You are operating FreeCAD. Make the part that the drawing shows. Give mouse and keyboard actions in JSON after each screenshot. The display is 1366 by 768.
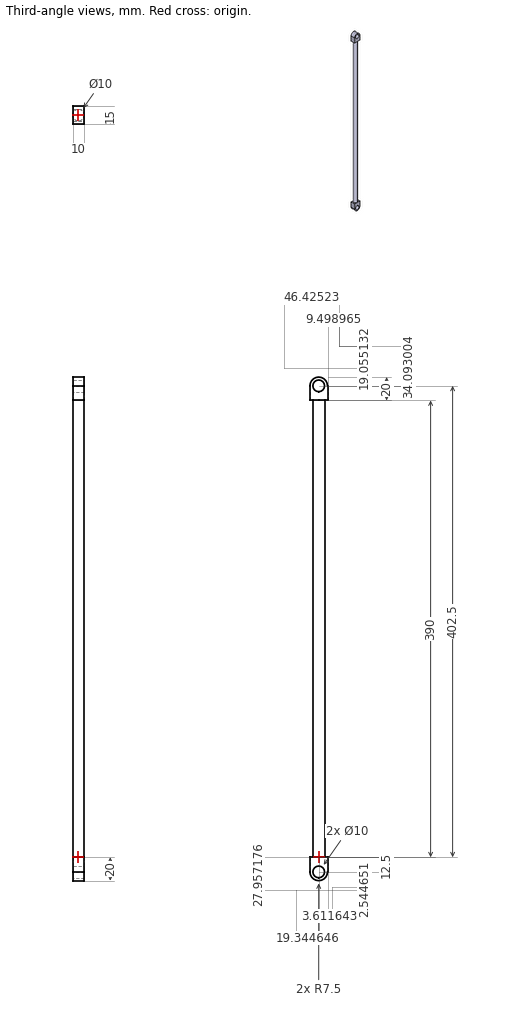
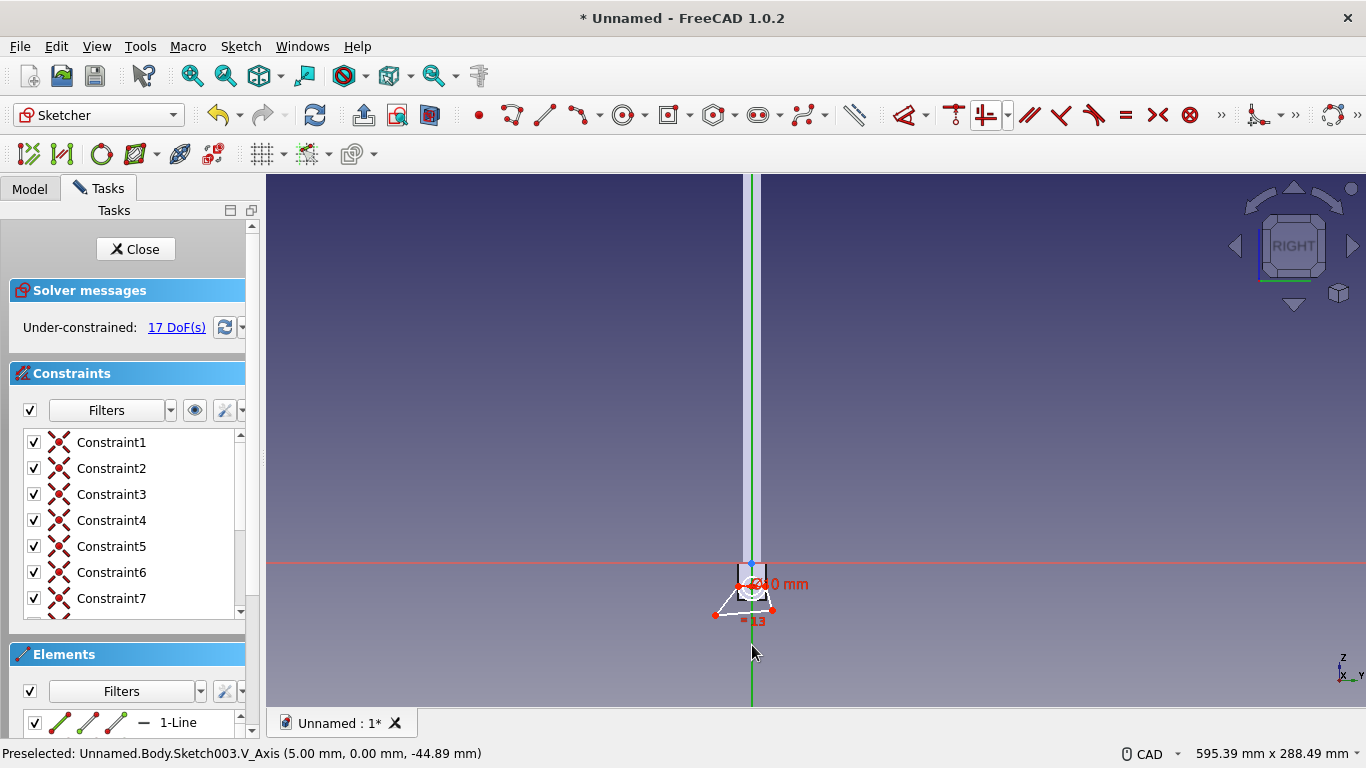
{"action": "left_click", "coordinate": [954, 116]}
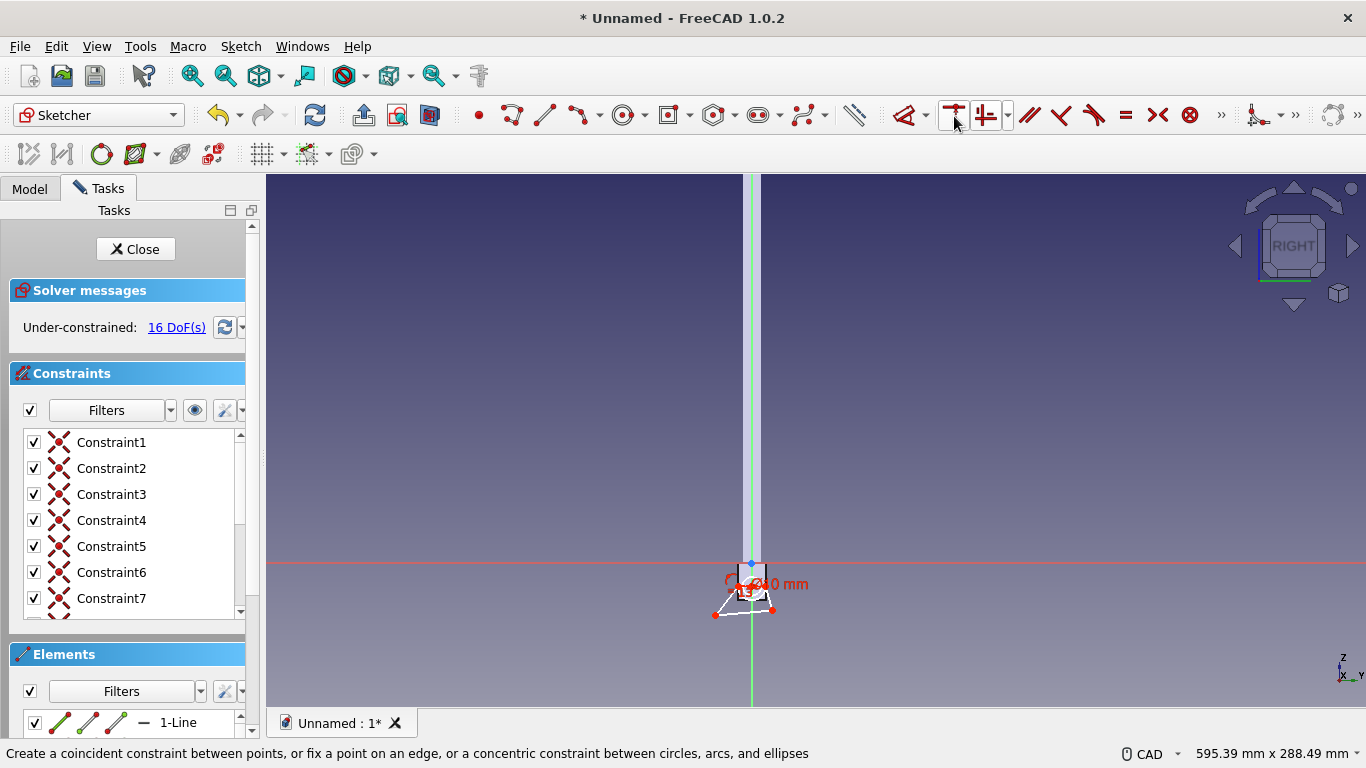
{"action": "scroll", "coordinate": [752, 589], "scroll_direction": "down", "scroll_amount": 5}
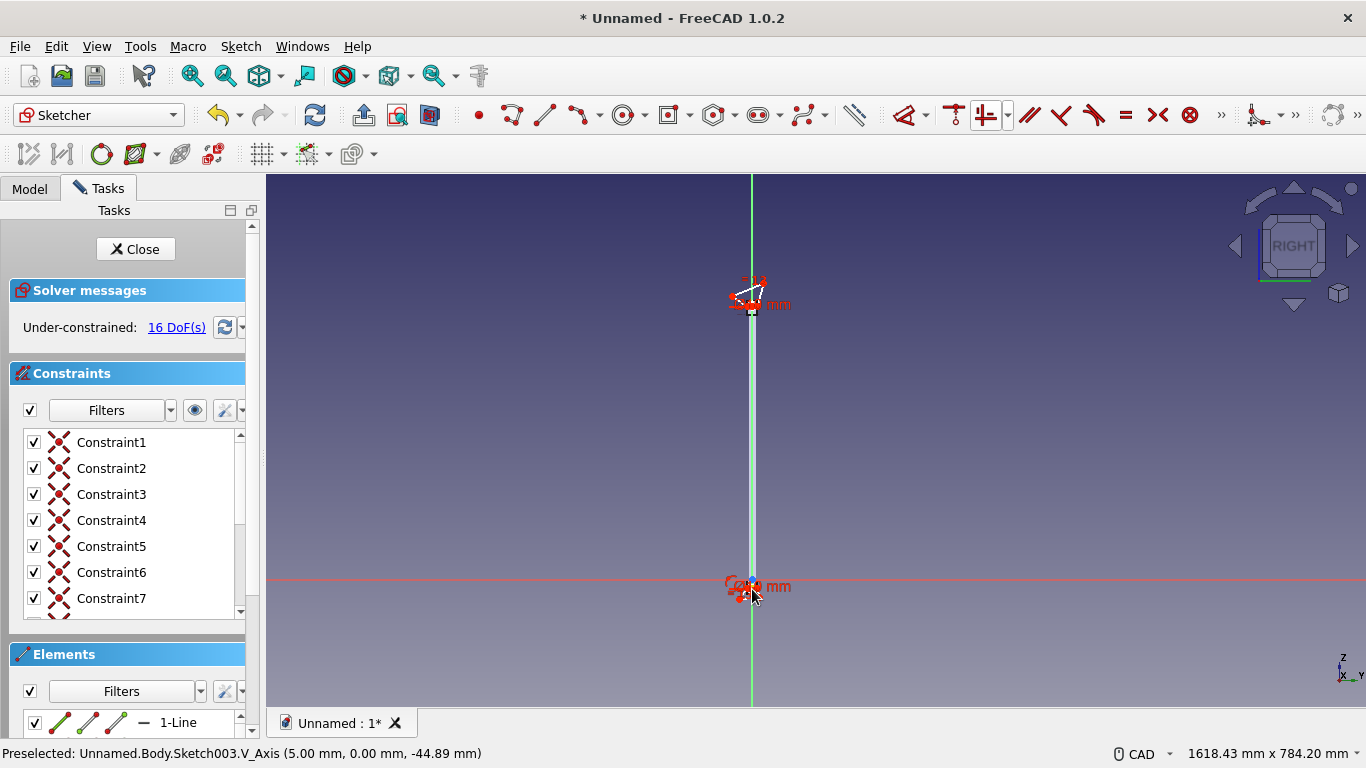
{"action": "scroll", "coordinate": [752, 307], "scroll_direction": "up", "scroll_amount": 5}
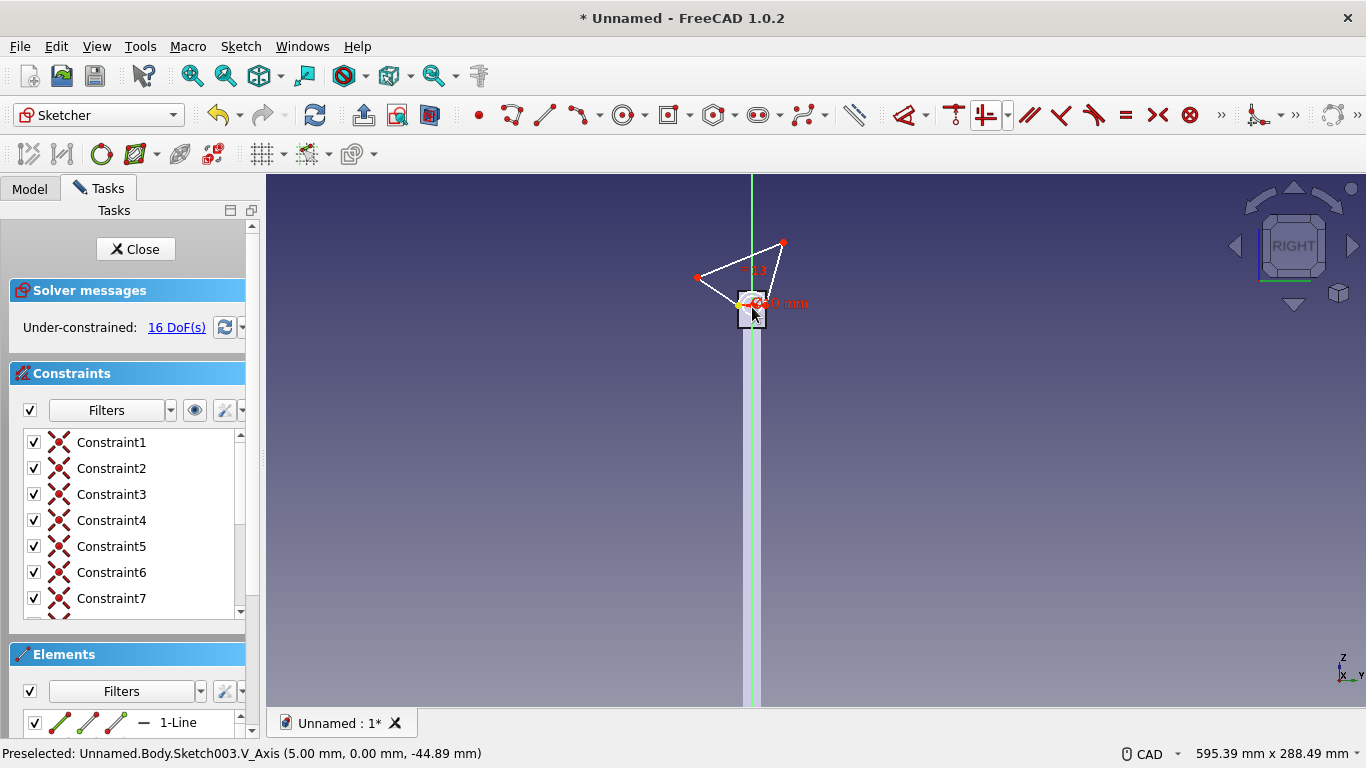
{"action": "left_click", "coordinate": [752, 305]}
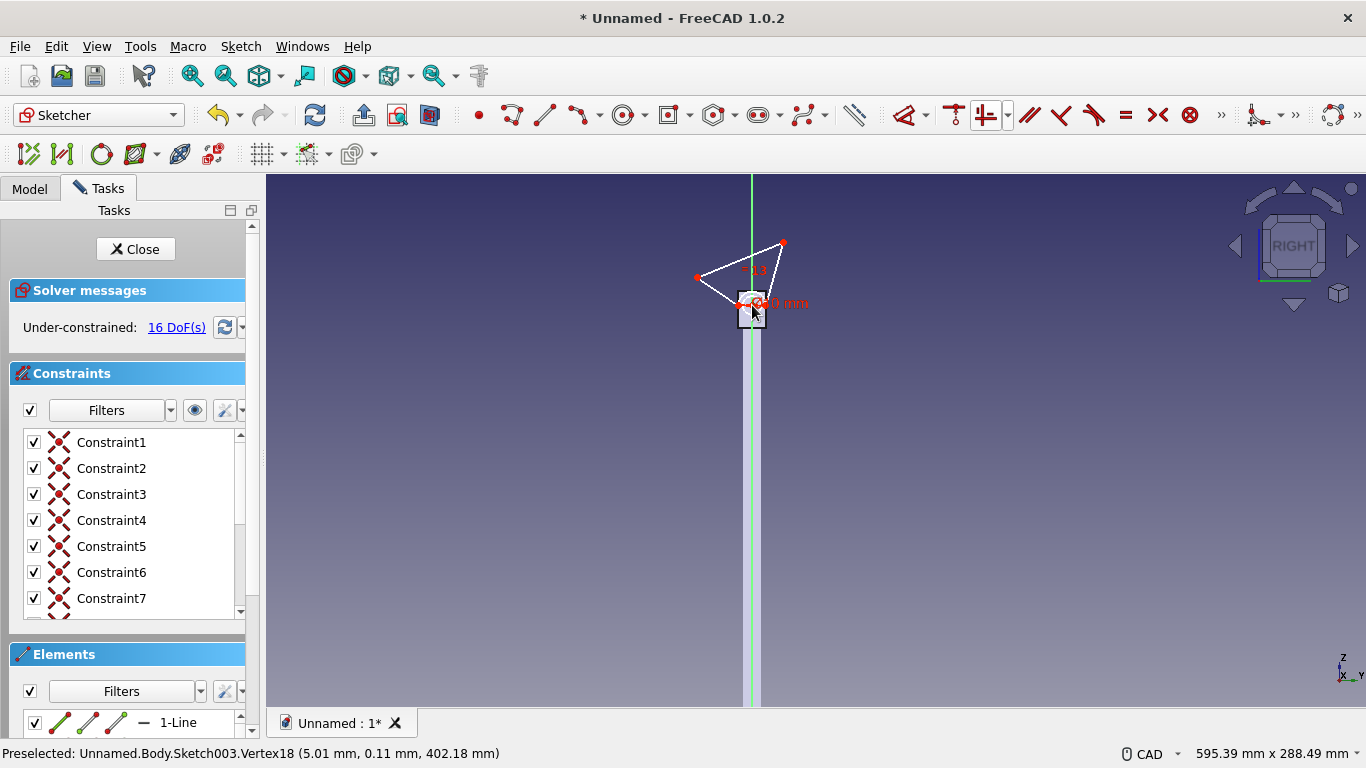
{"action": "left_click", "coordinate": [752, 645]}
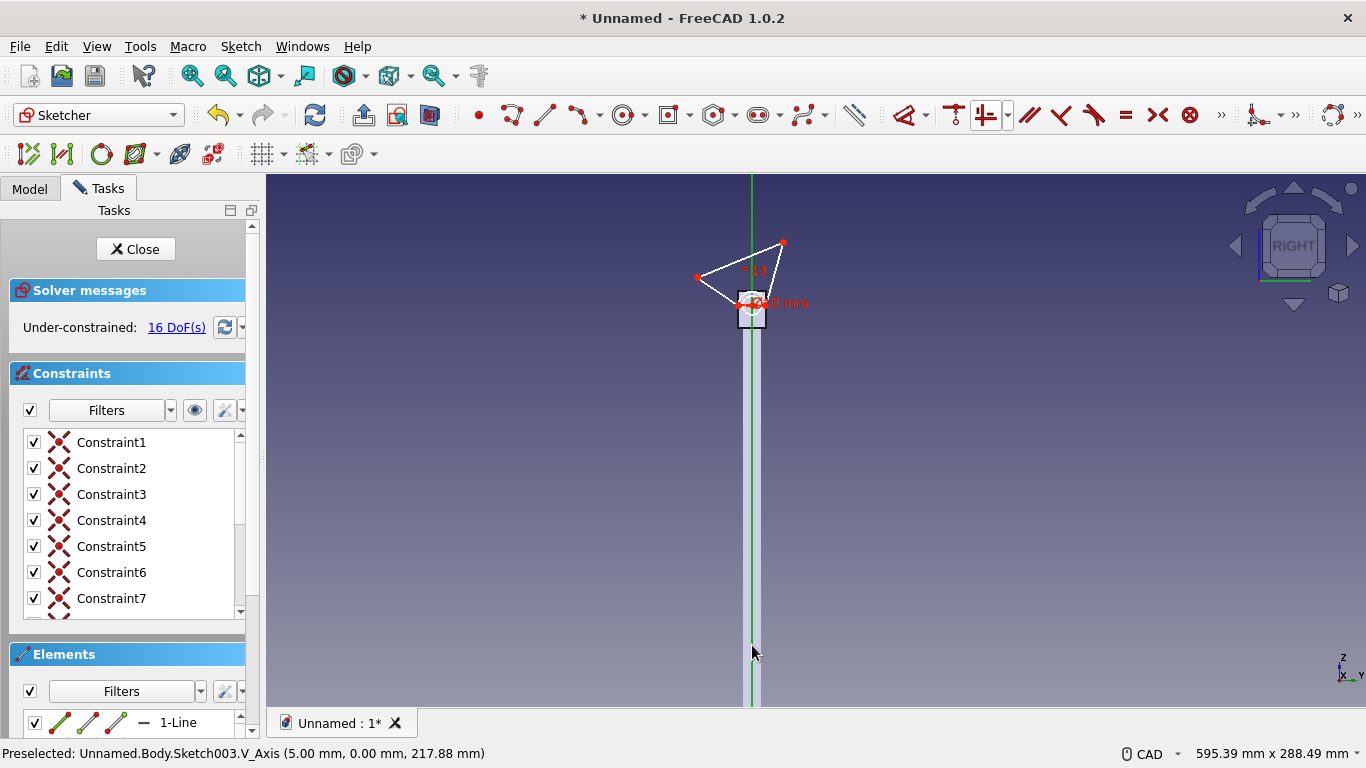
{"action": "left_click", "coordinate": [954, 116]}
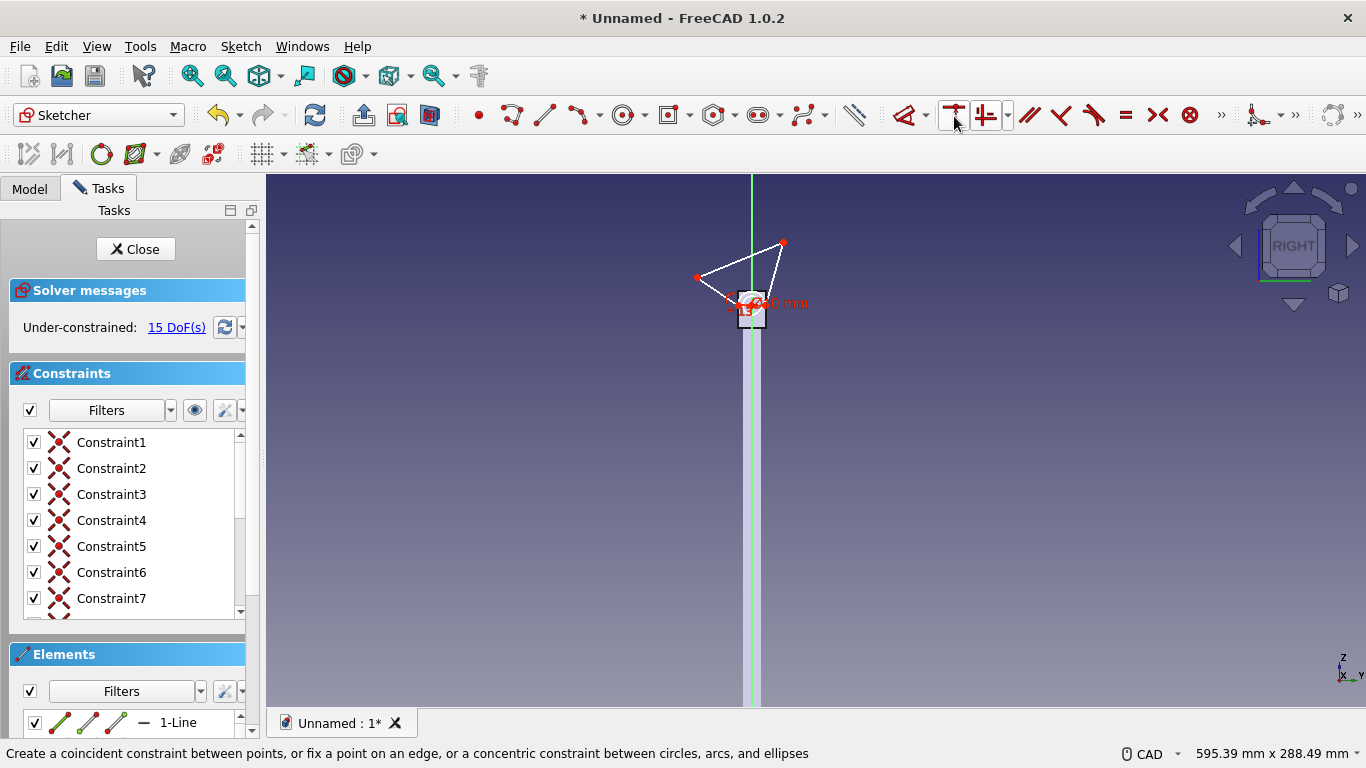
{"action": "left_click", "coordinate": [904, 116]}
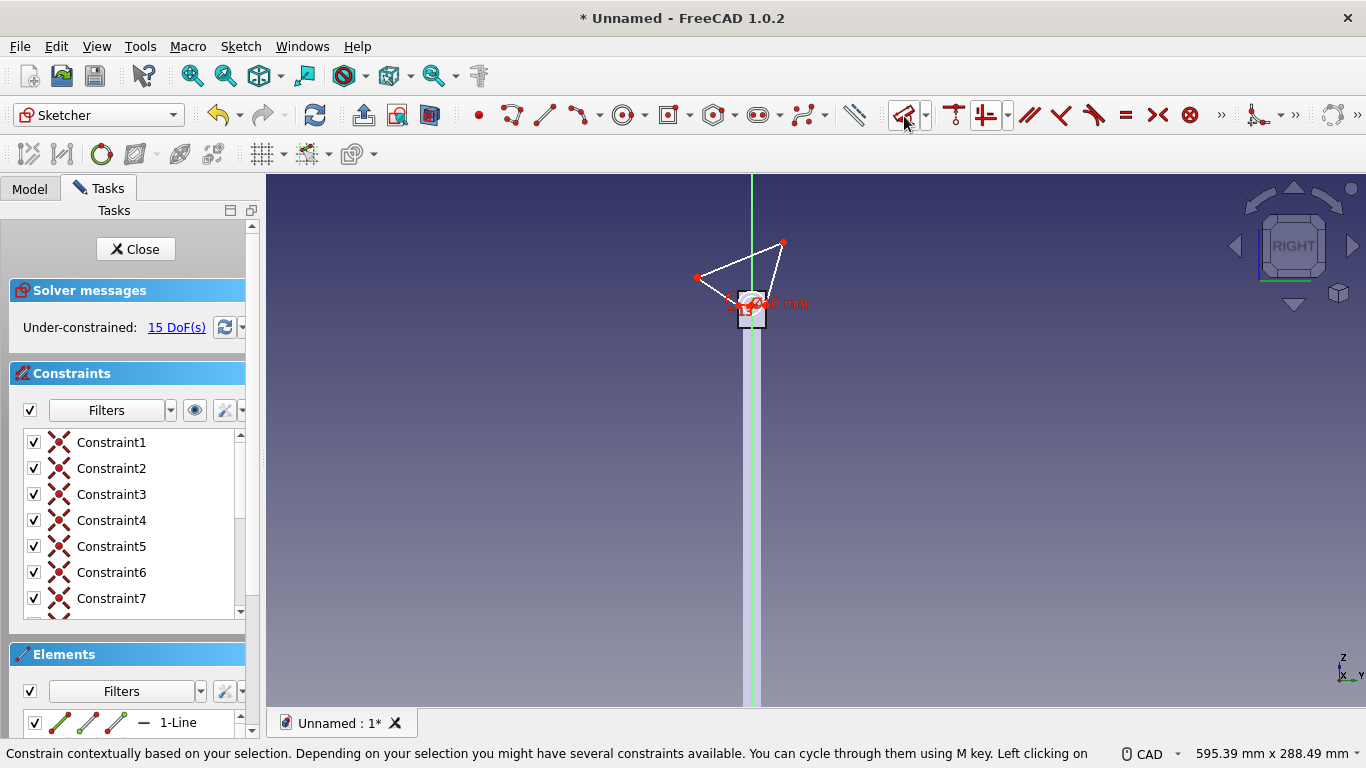
{"action": "scroll", "coordinate": [752, 306], "scroll_direction": "down", "scroll_amount": 5}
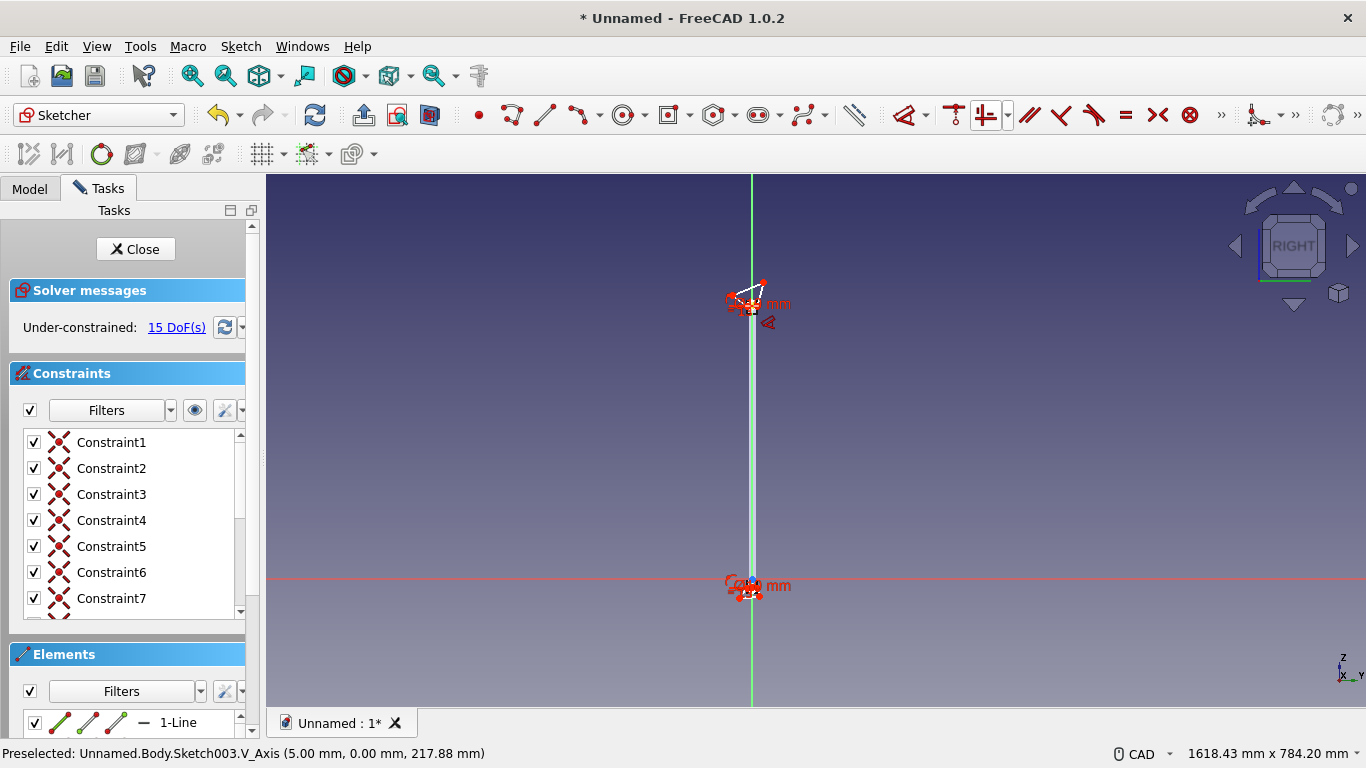
{"action": "scroll", "coordinate": [755, 592], "scroll_direction": "up", "scroll_amount": 11}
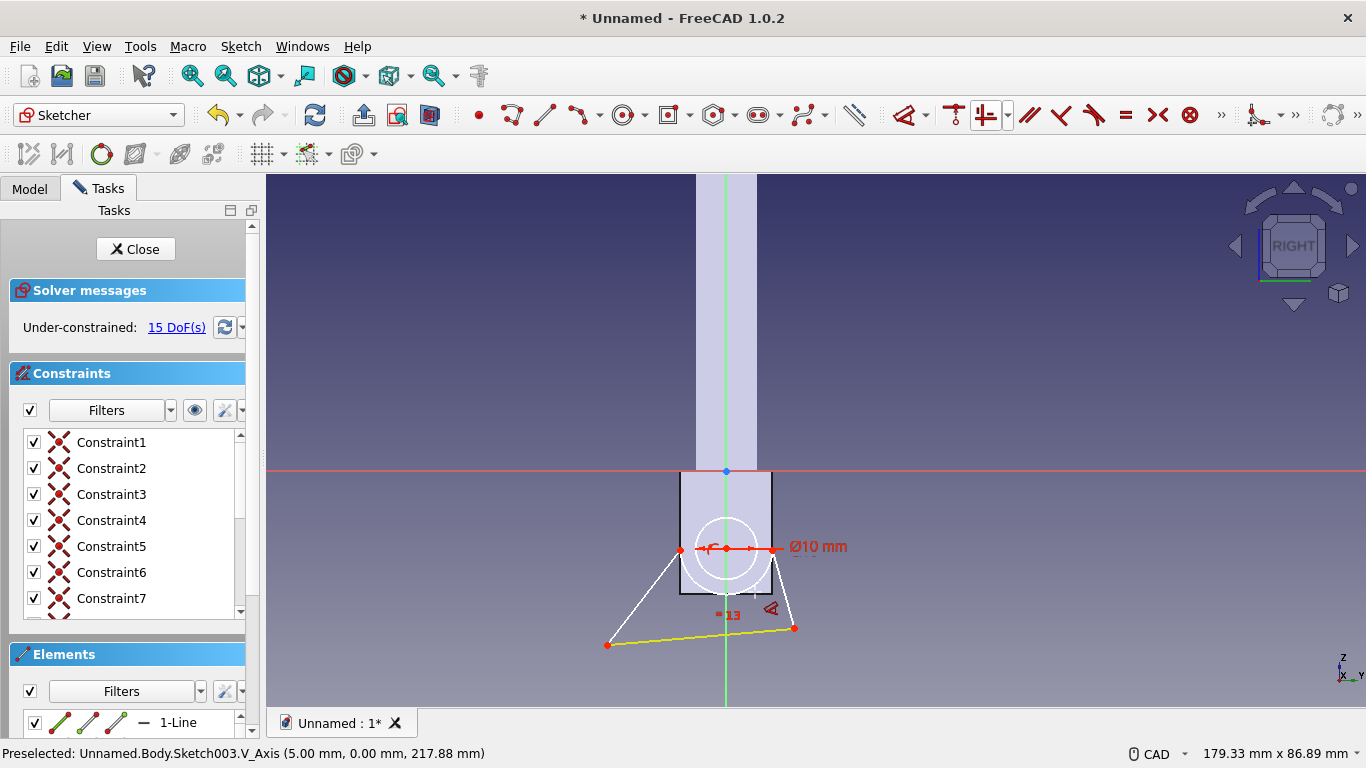
{"action": "left_click", "coordinate": [753, 586]}
{"action": "left_click", "coordinate": [771, 612]}